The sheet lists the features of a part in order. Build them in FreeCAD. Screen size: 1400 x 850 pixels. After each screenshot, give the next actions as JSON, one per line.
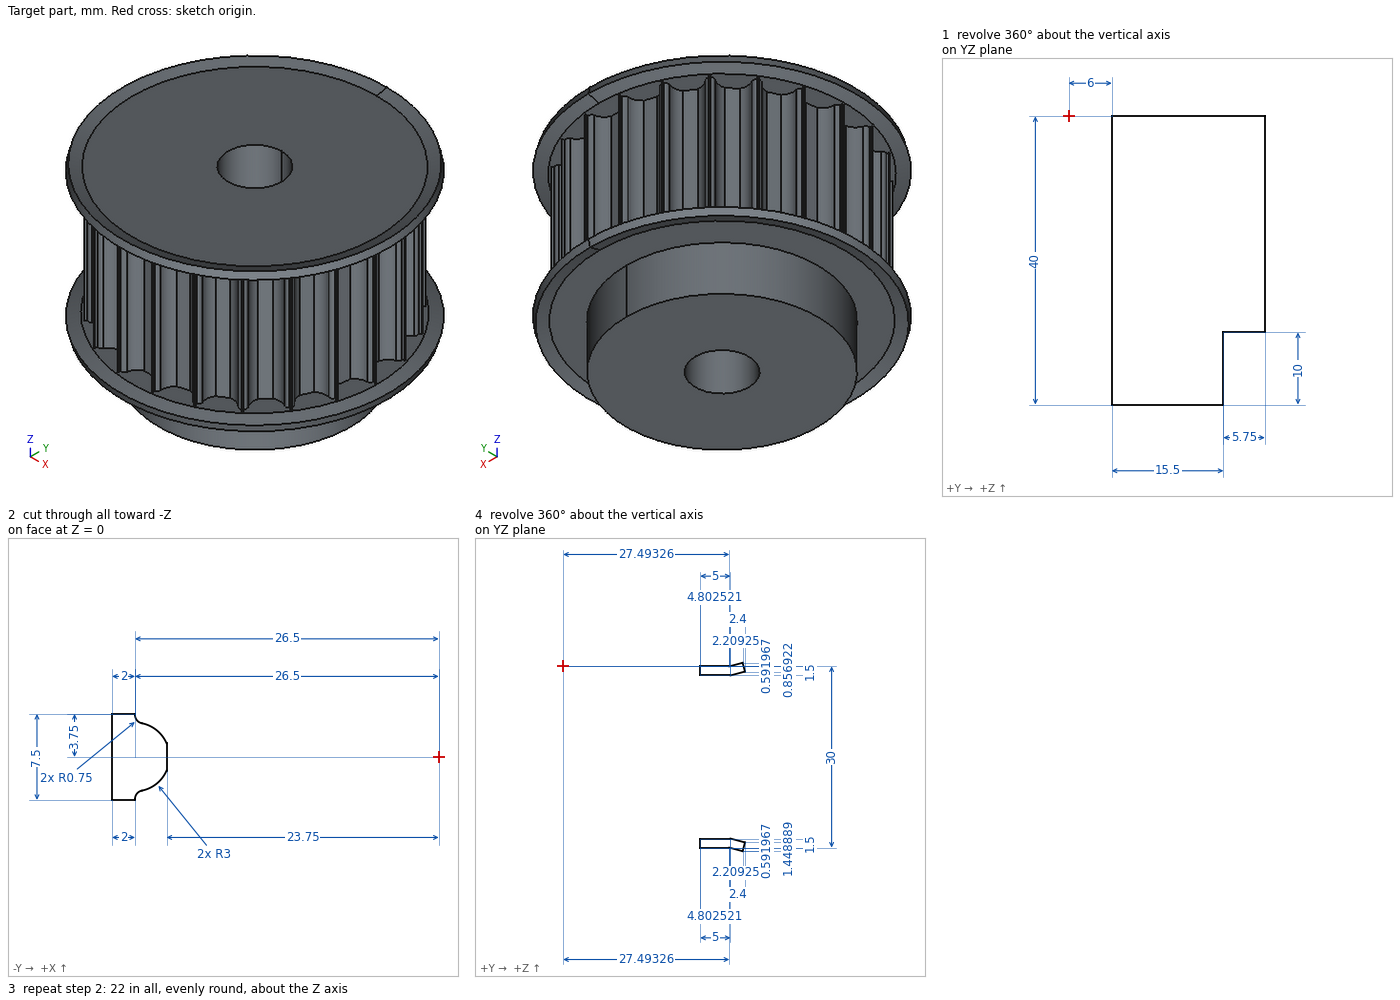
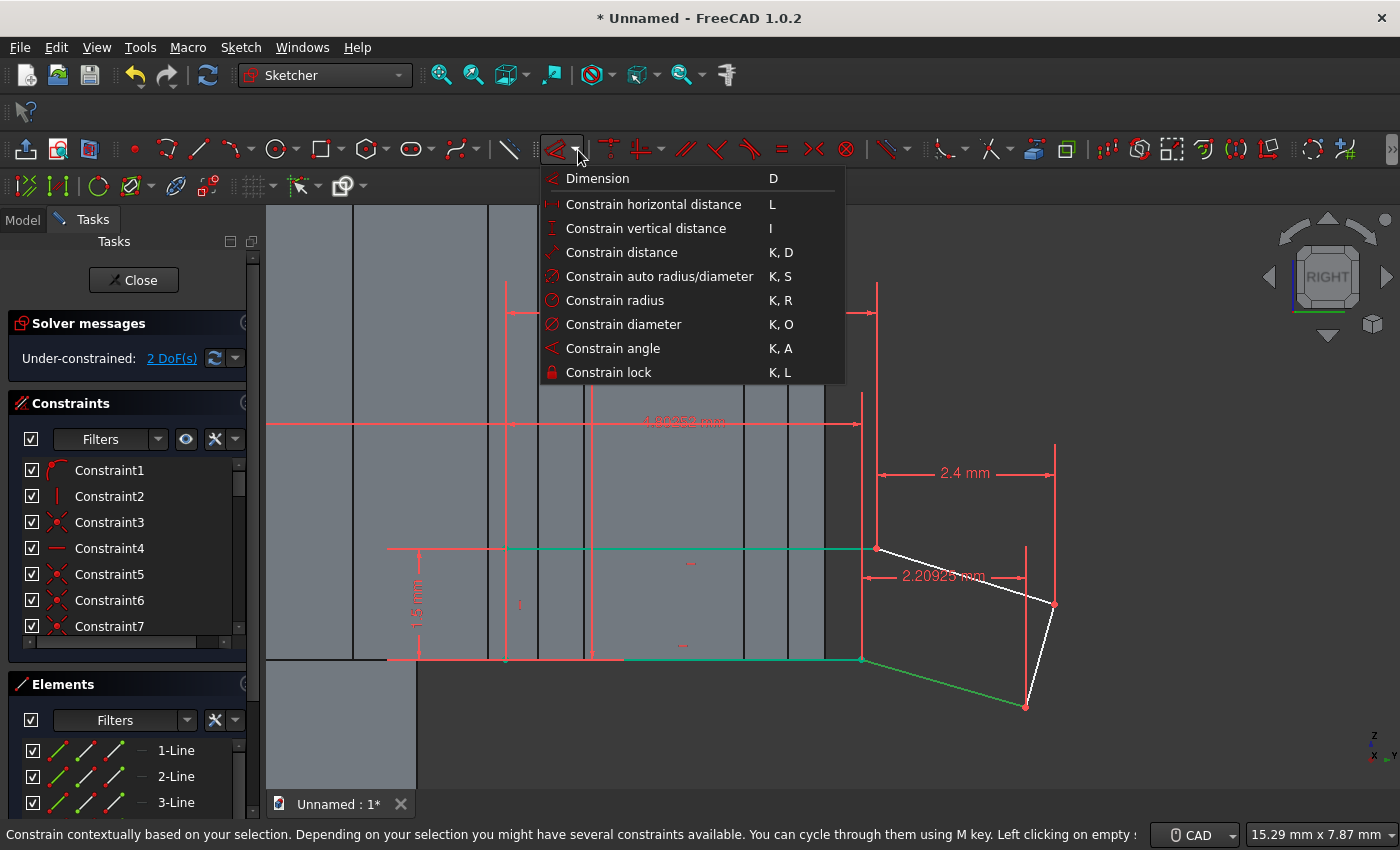
{"action": "left_click", "coordinate": [693, 228]}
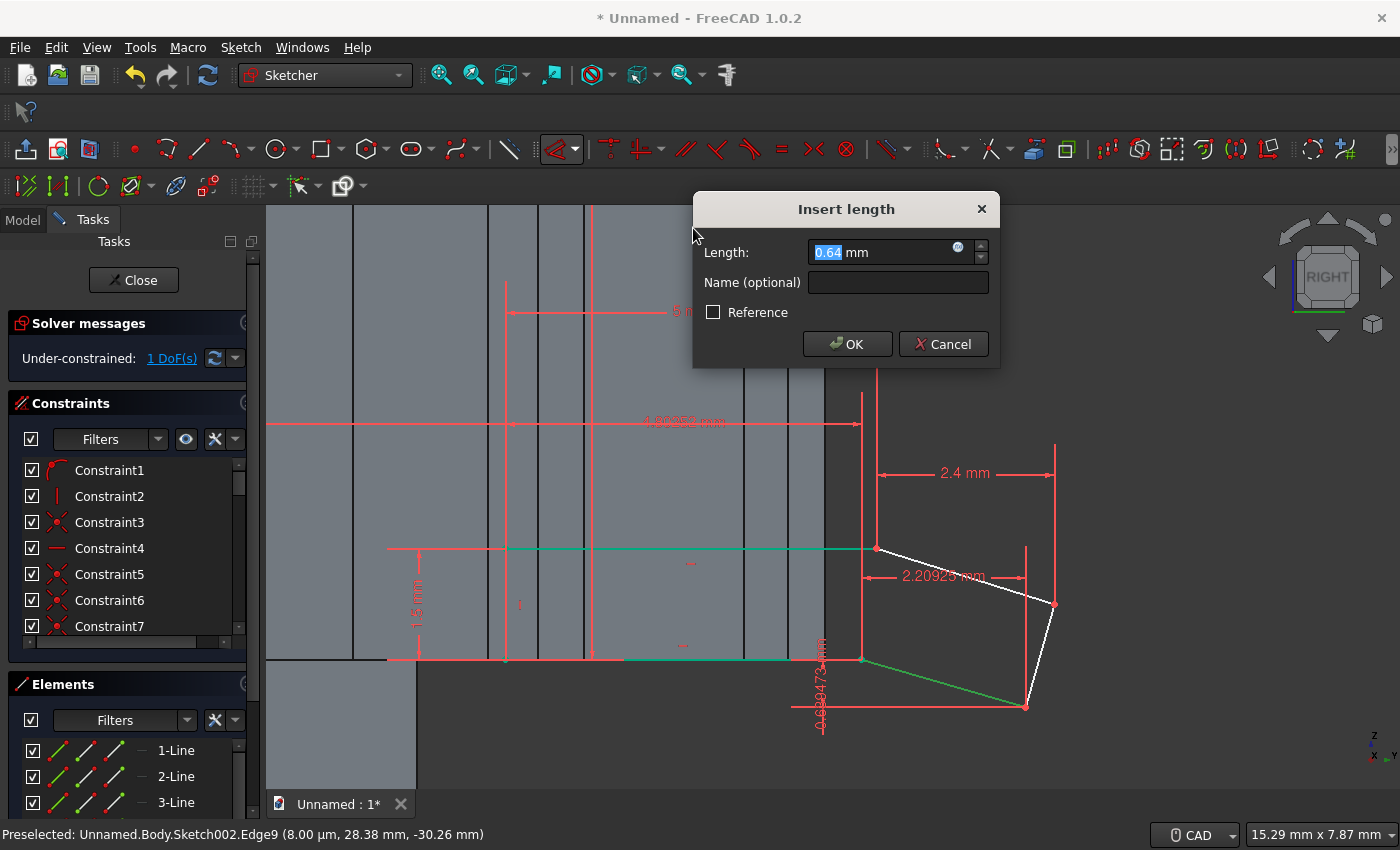
{"action": "type", "text": "0.591967"}
{"action": "key", "text": "Return"}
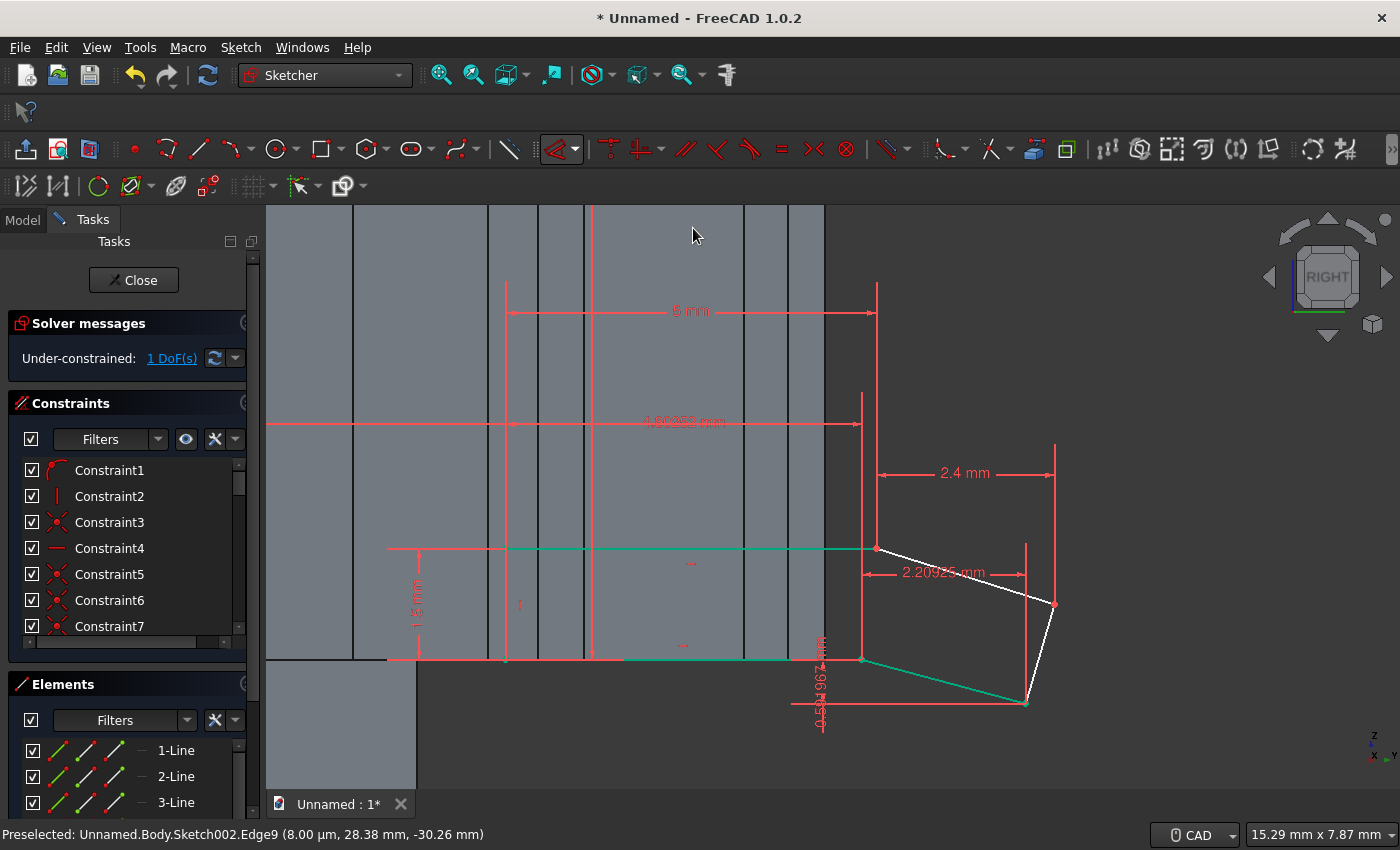
{"action": "left_click", "coordinate": [1034, 674]}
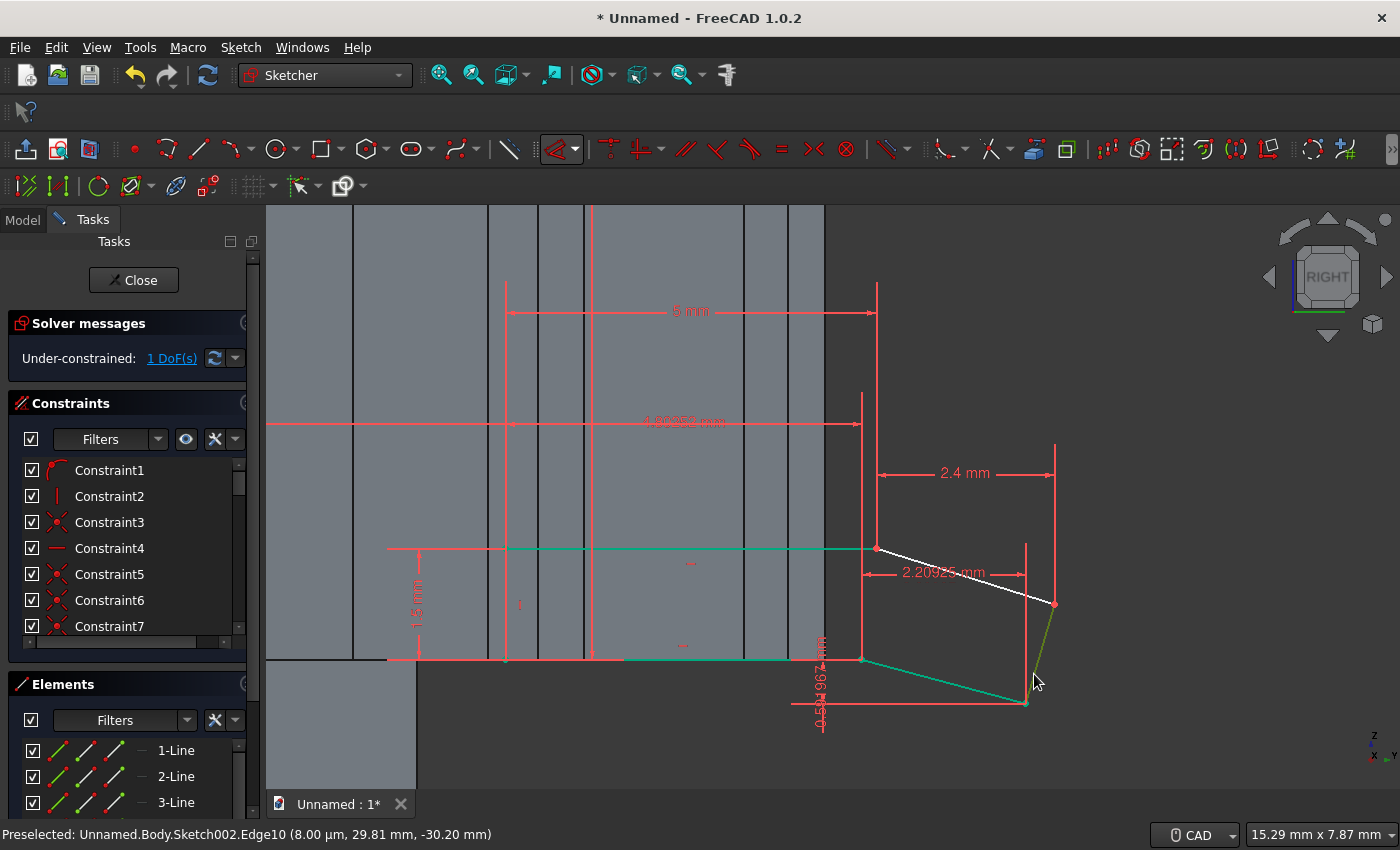
{"action": "left_click", "coordinate": [578, 150]}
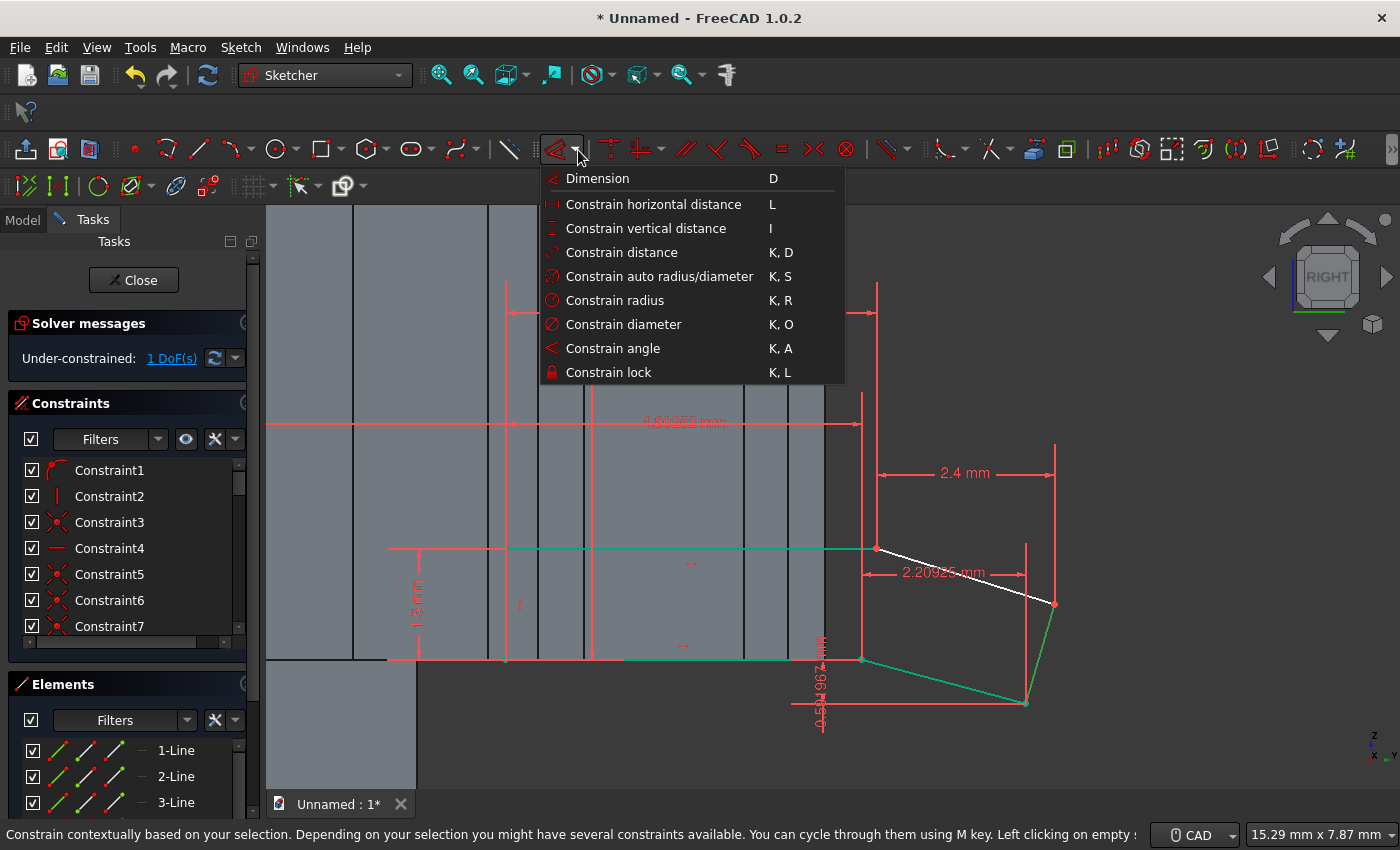
{"action": "left_click", "coordinate": [693, 228]}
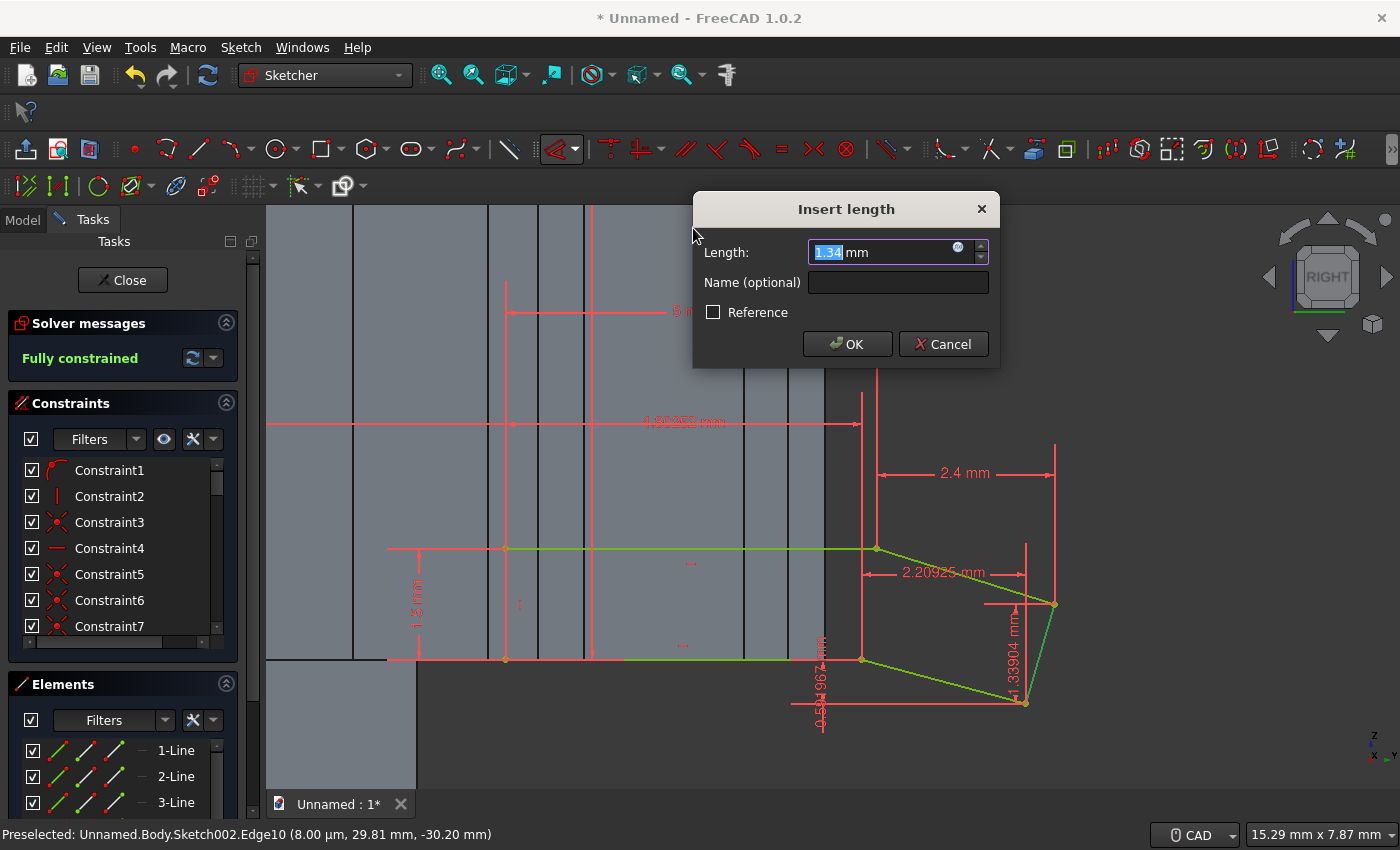
{"action": "type", "text": "1.448889"}
{"action": "key", "text": "Return"}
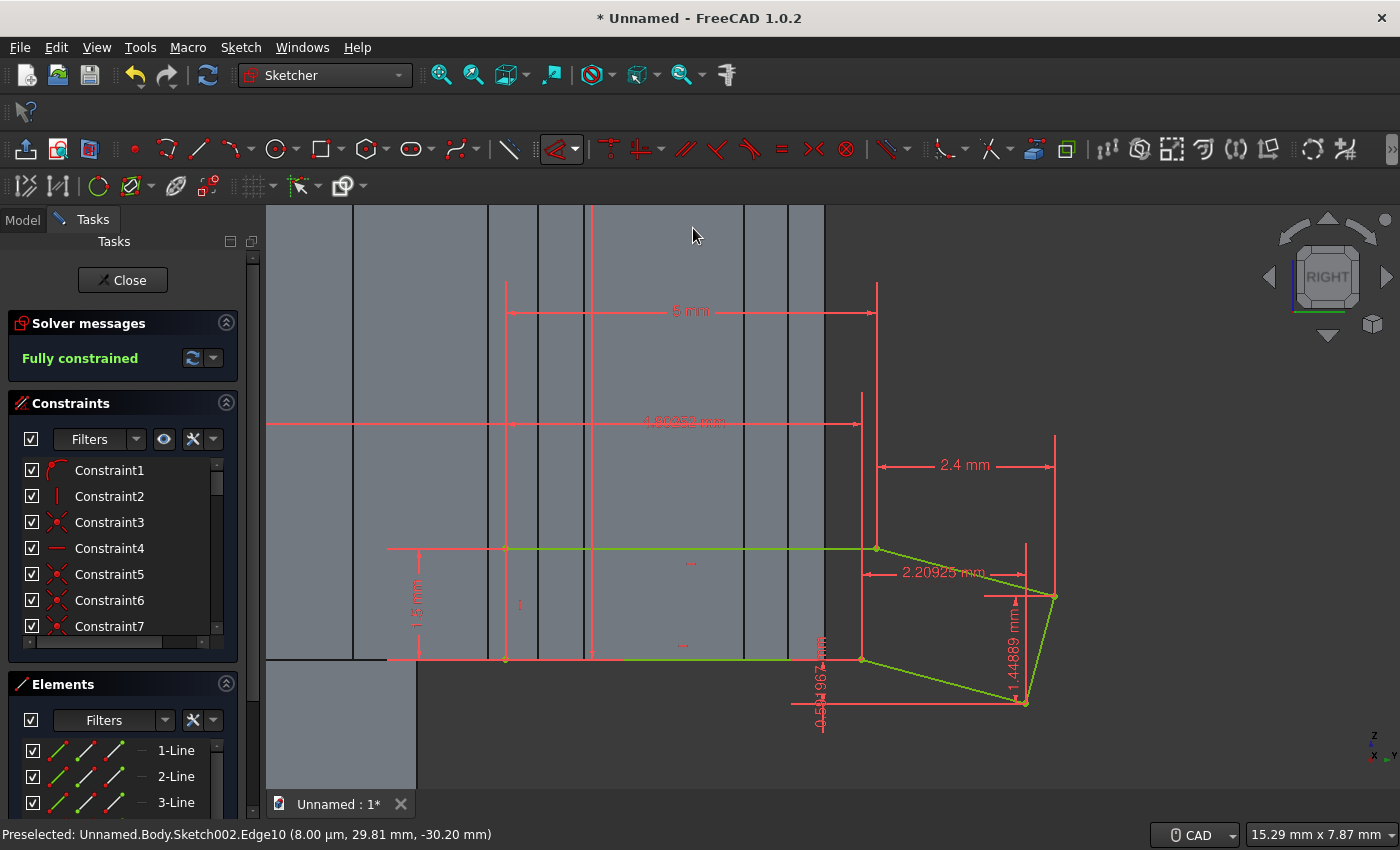
{"action": "left_click", "coordinate": [123, 280]}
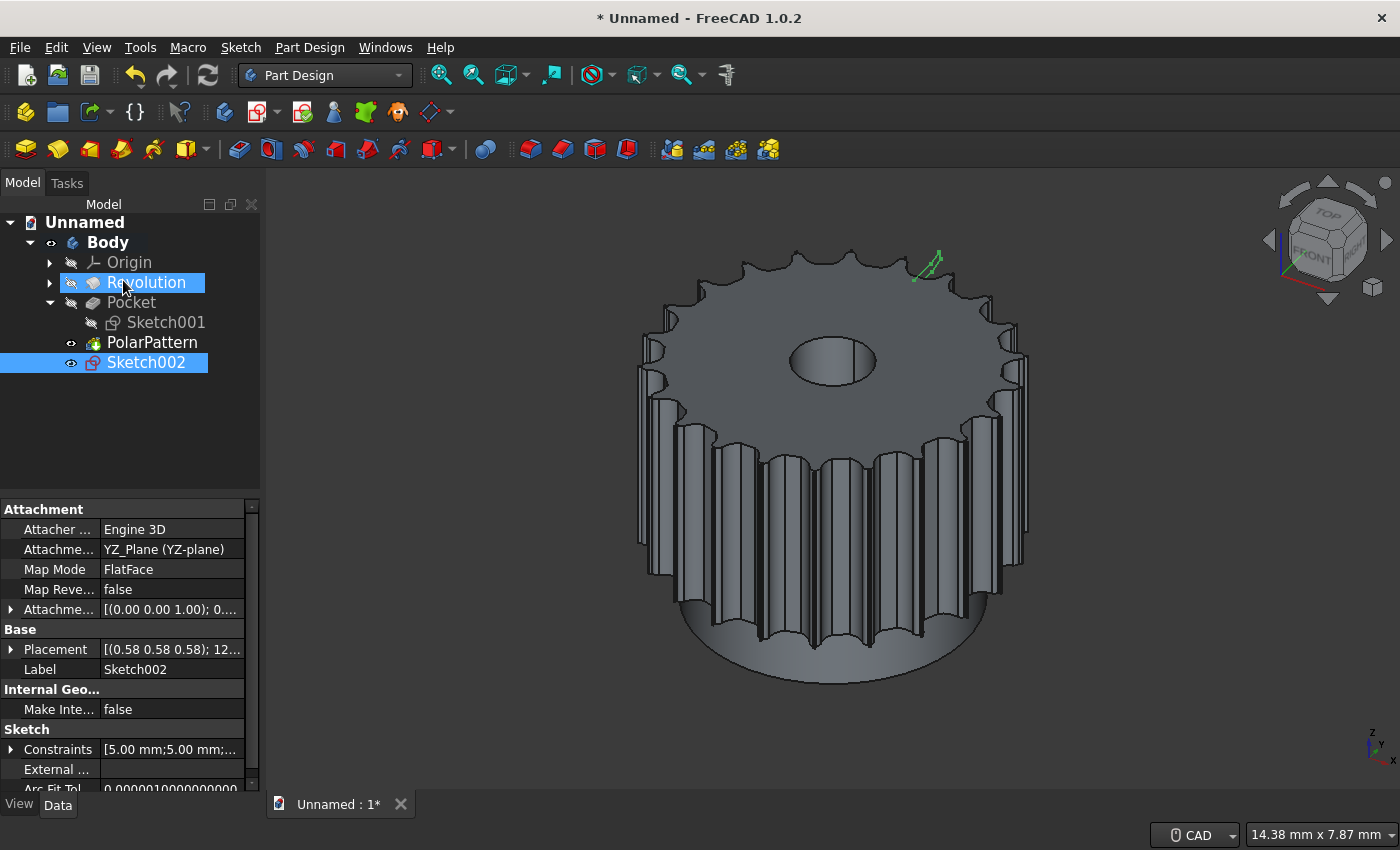
{"action": "left_click", "coordinate": [58, 150]}